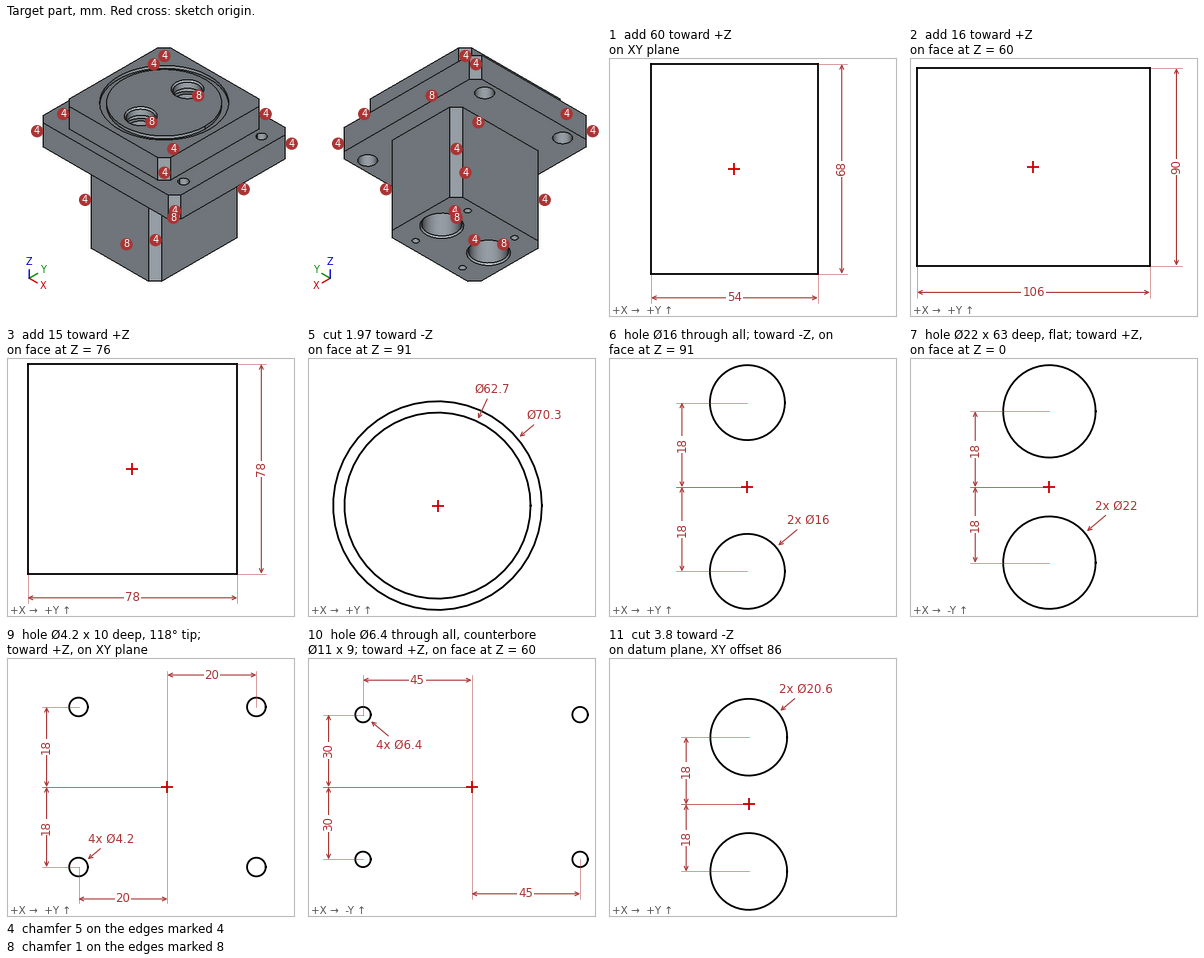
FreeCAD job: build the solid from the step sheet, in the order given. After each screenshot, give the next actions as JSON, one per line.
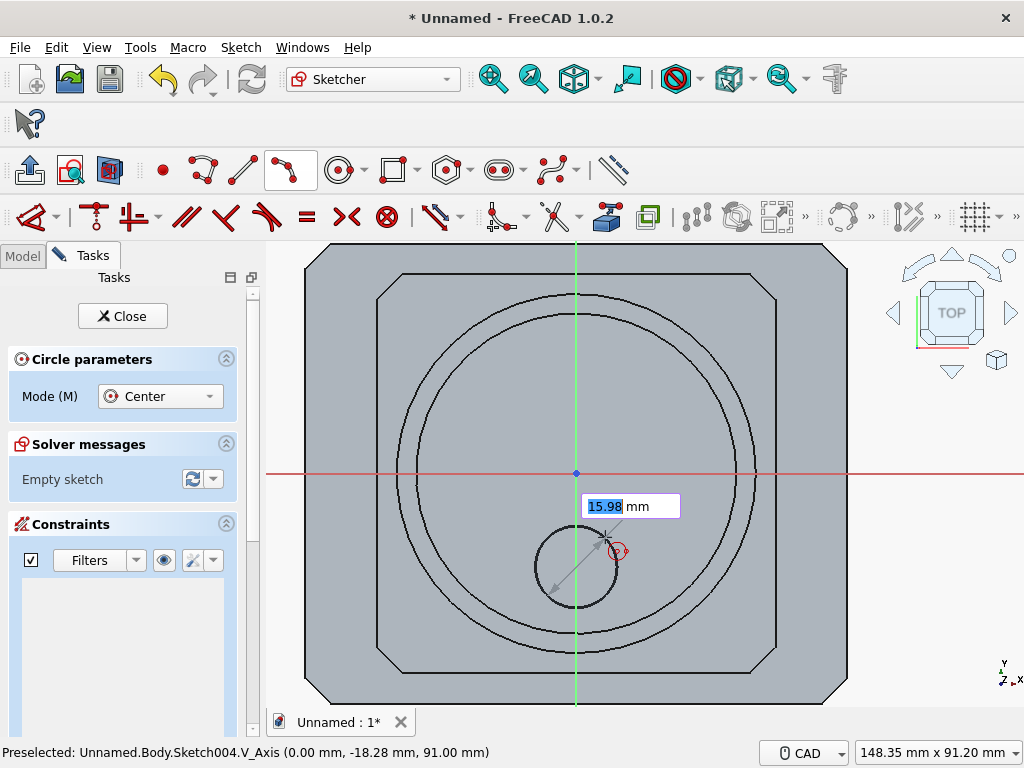
{"action": "type", "text": "16"}
{"action": "key", "text": "Return"}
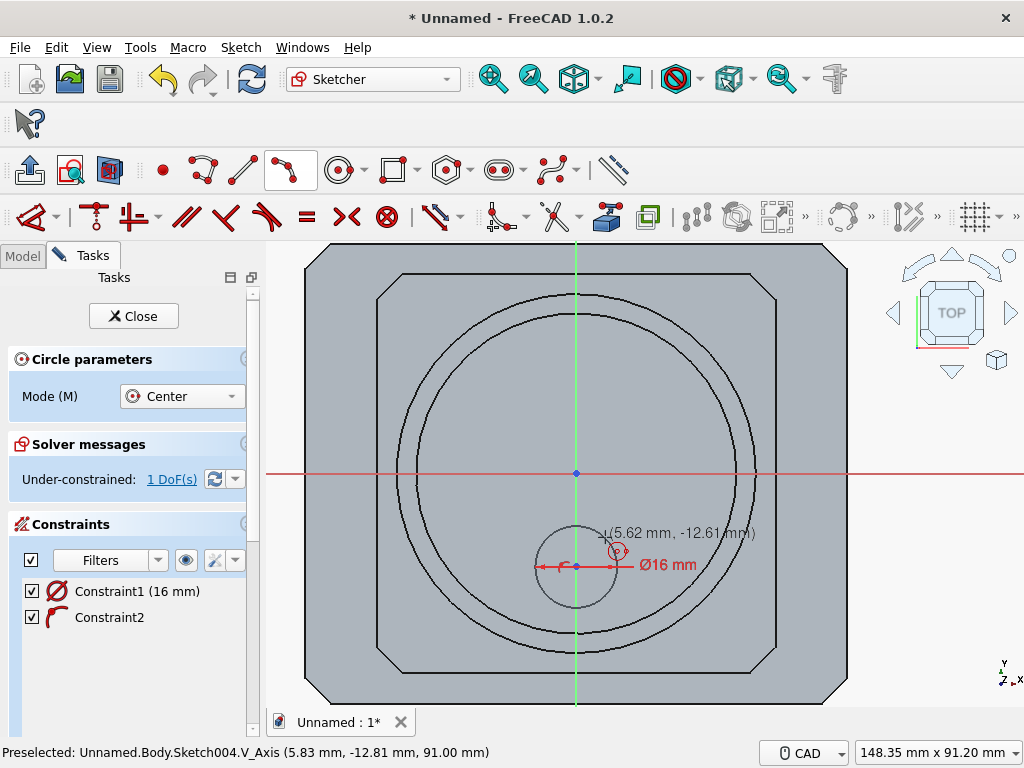
{"action": "left_click", "coordinate": [576, 382]}
{"action": "mouse_move", "coordinate": [605, 353]}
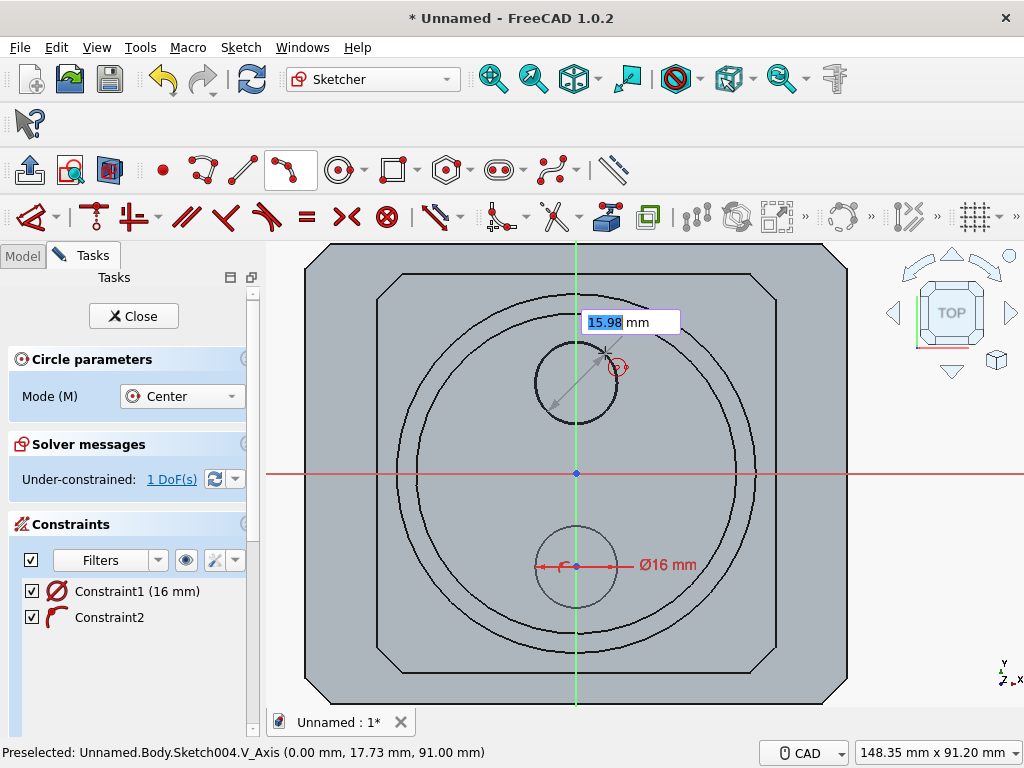
{"action": "type", "text": "16"}
{"action": "key", "text": "Return"}
{"action": "key", "text": "Escape"}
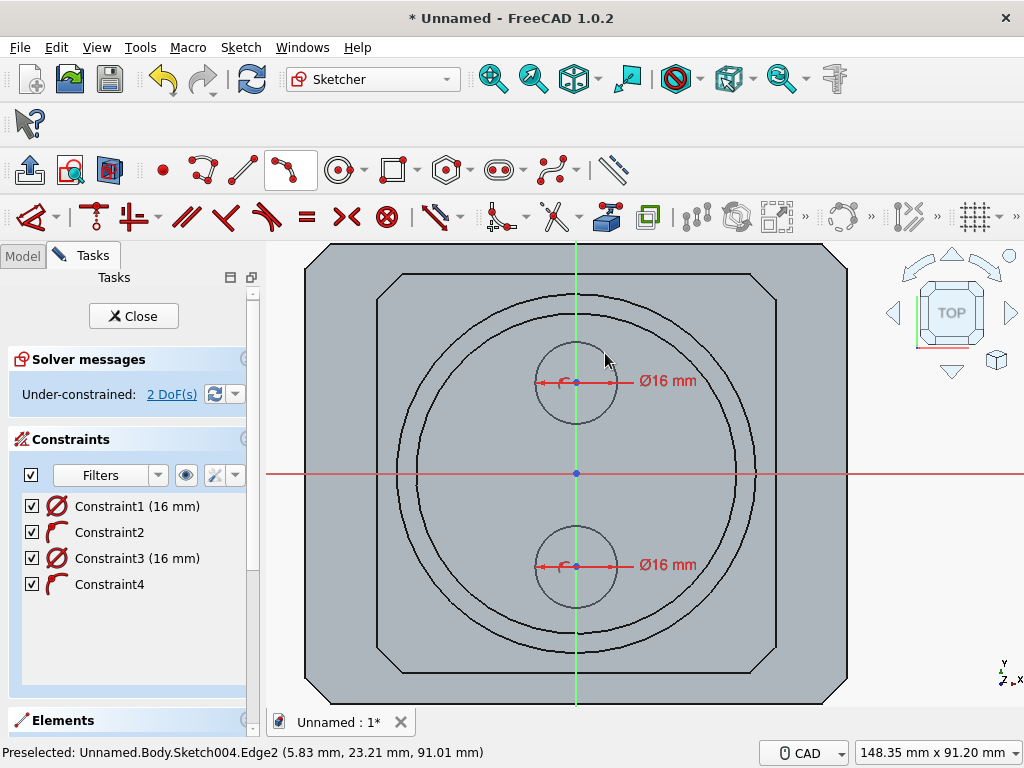
{"action": "key", "text": "d"}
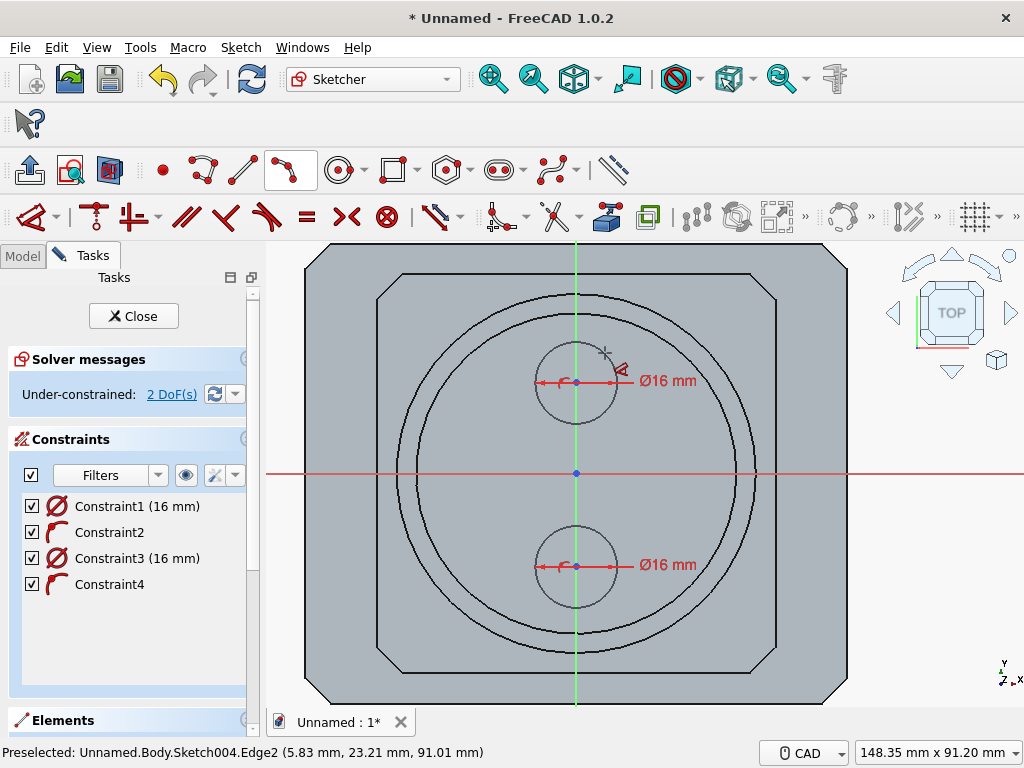
{"action": "left_click", "coordinate": [576, 567]}
{"action": "left_click", "coordinate": [610, 520]}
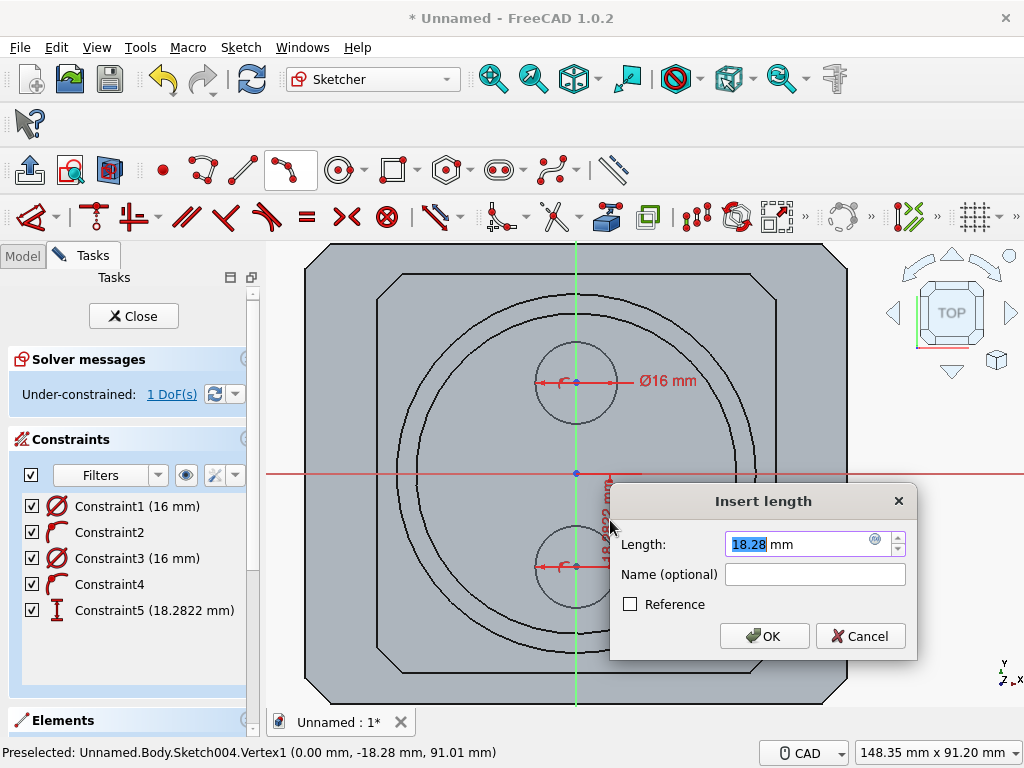
{"action": "type", "text": "18"}
{"action": "key", "text": "Return"}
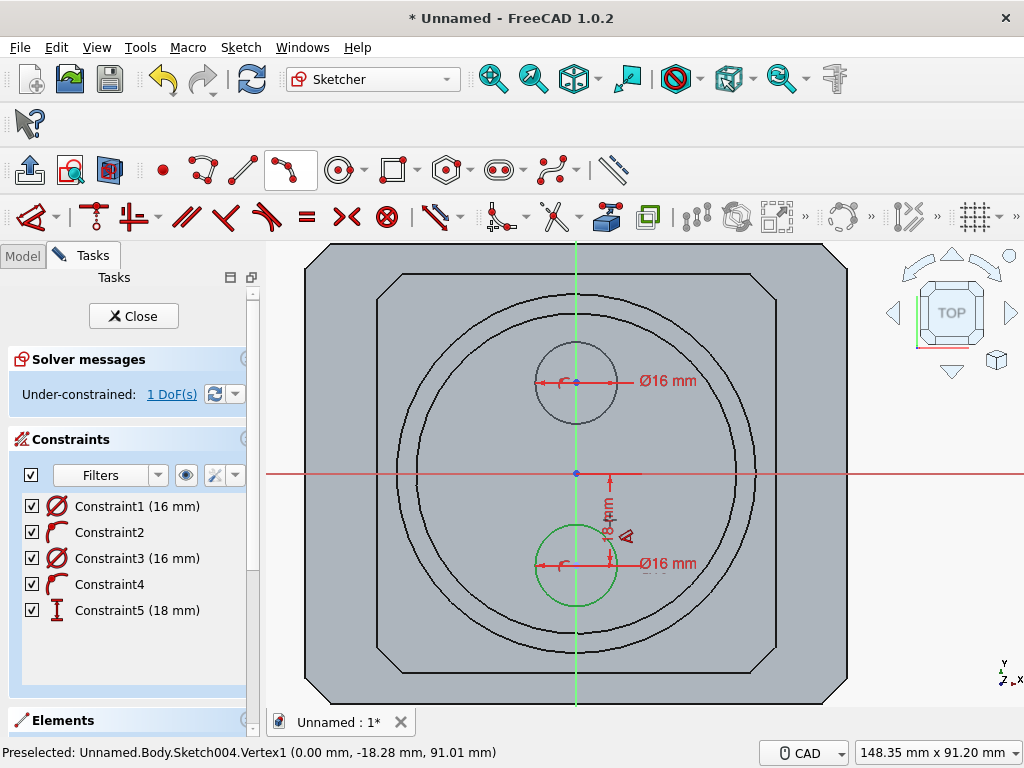
{"action": "left_click", "coordinate": [576, 383]}
{"action": "left_click", "coordinate": [610, 428]}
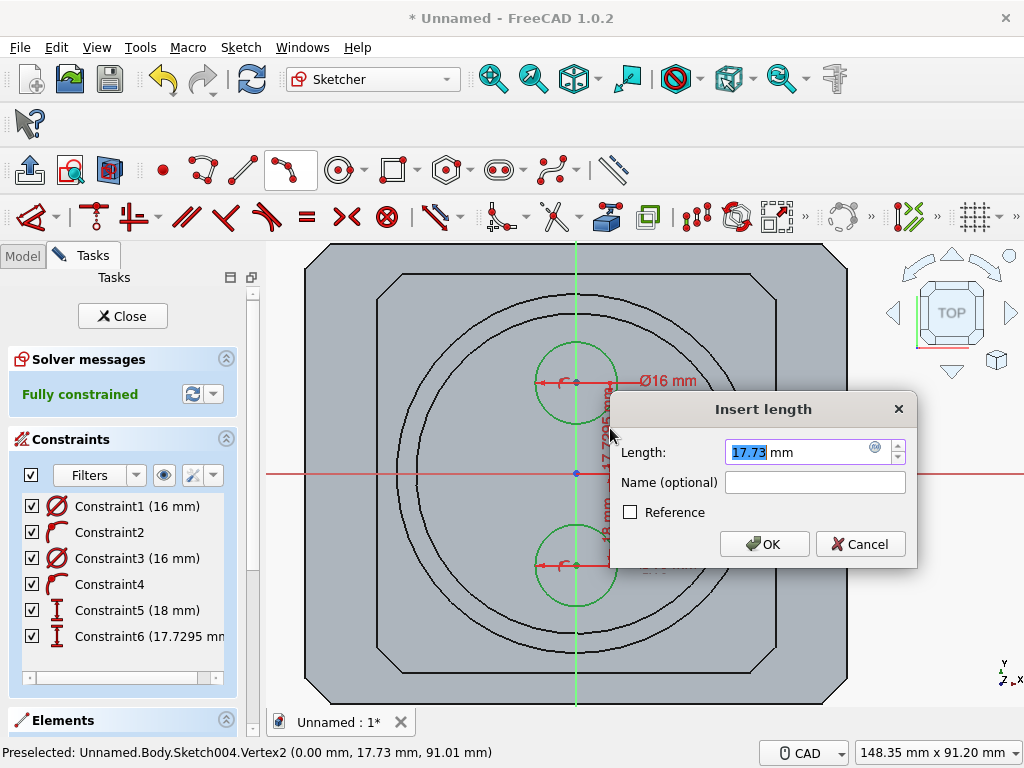
{"action": "type", "text": "18"}
{"action": "key", "text": "Return"}
{"action": "key", "text": "Escape"}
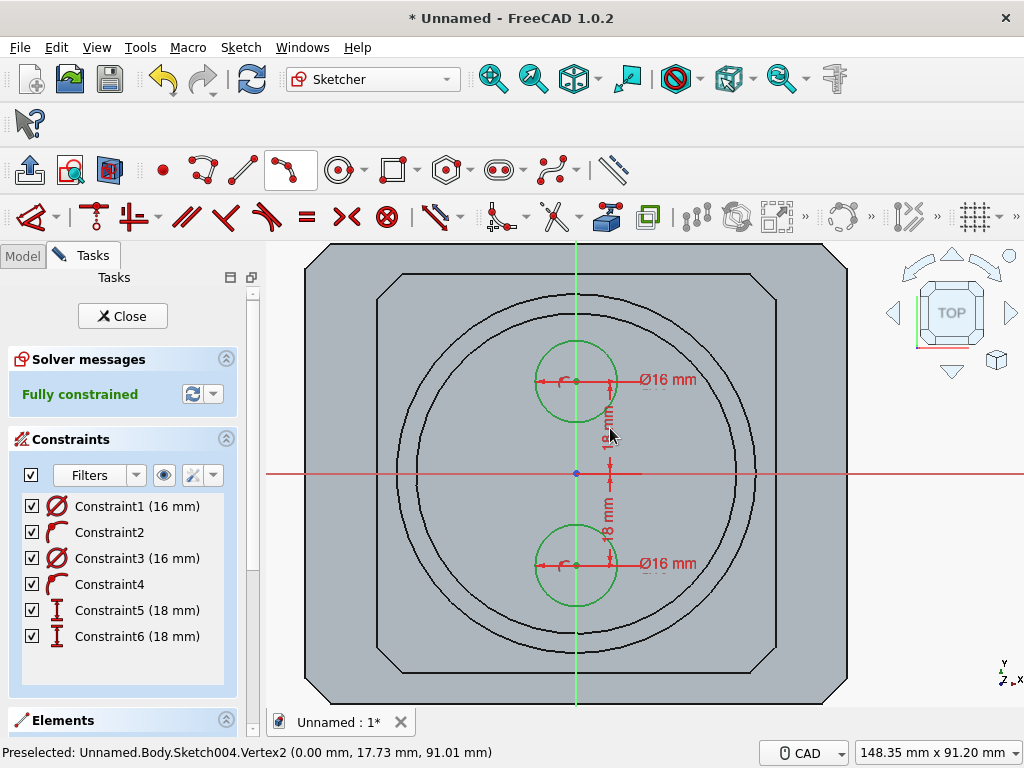
{"action": "left_click", "coordinate": [123, 316]}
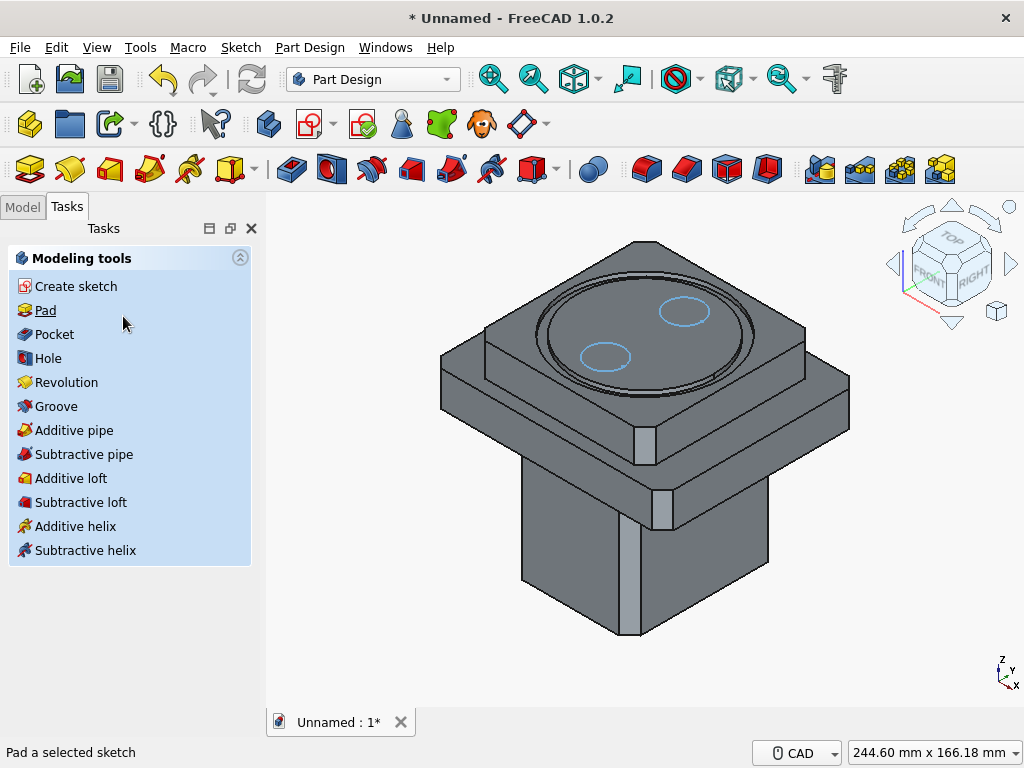
{"action": "left_click", "coordinate": [332, 170]}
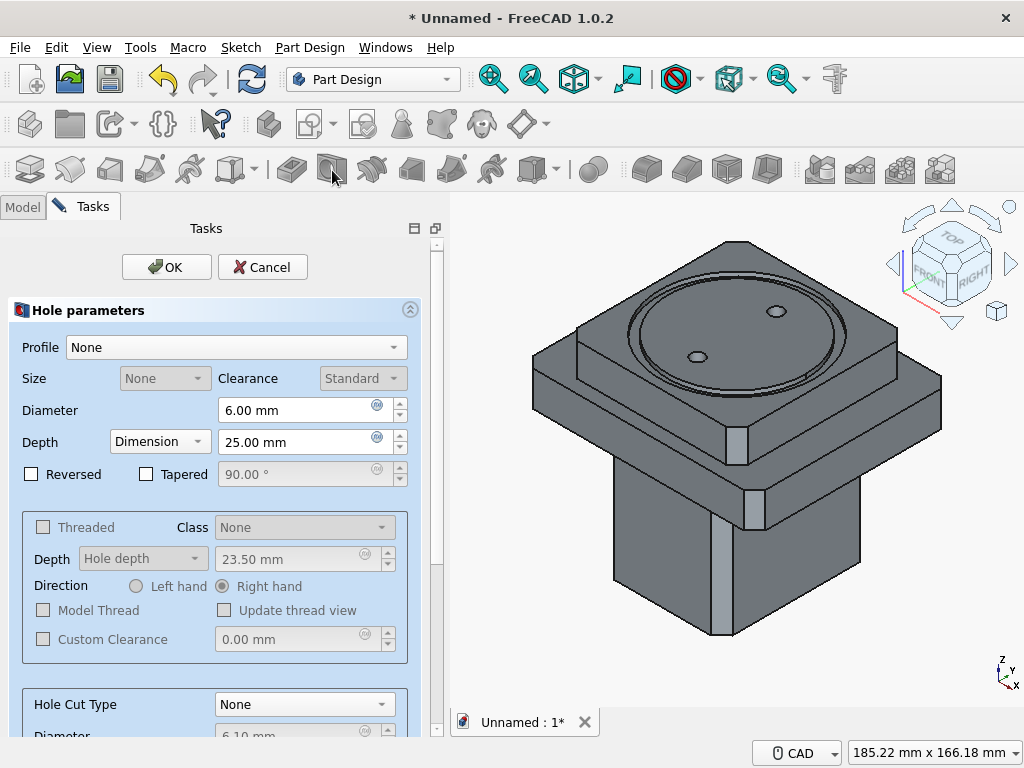
{"action": "triple_click", "coordinate": [305, 410]}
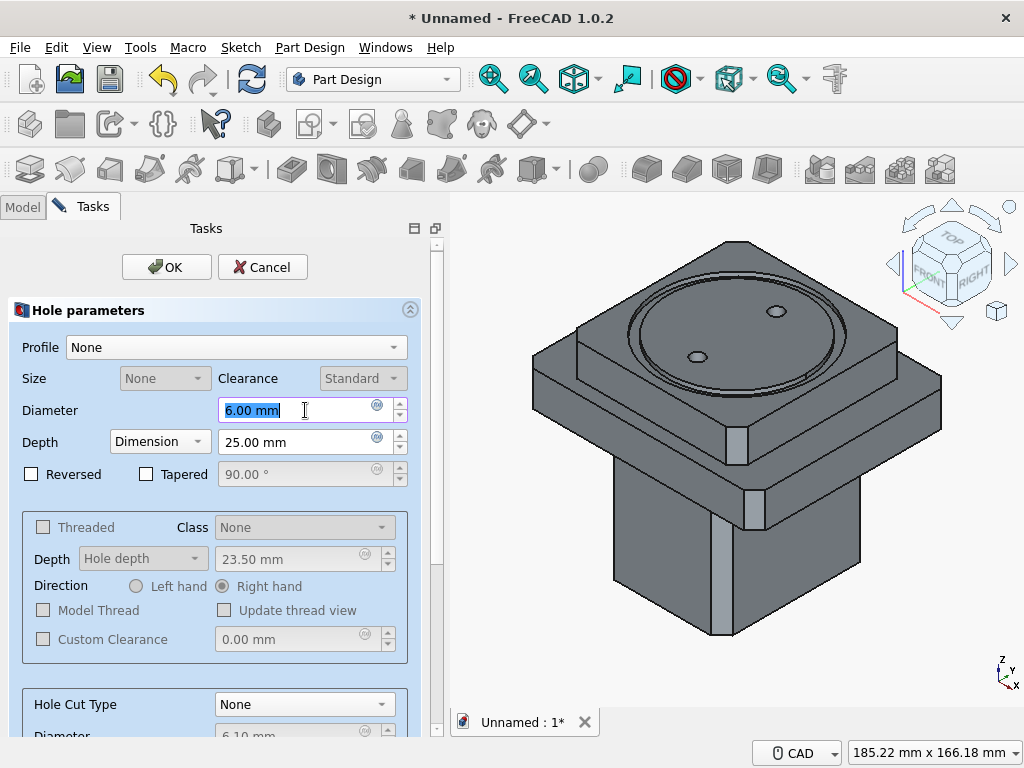
{"action": "type", "text": "16"}
{"action": "key", "text": "Tab"}